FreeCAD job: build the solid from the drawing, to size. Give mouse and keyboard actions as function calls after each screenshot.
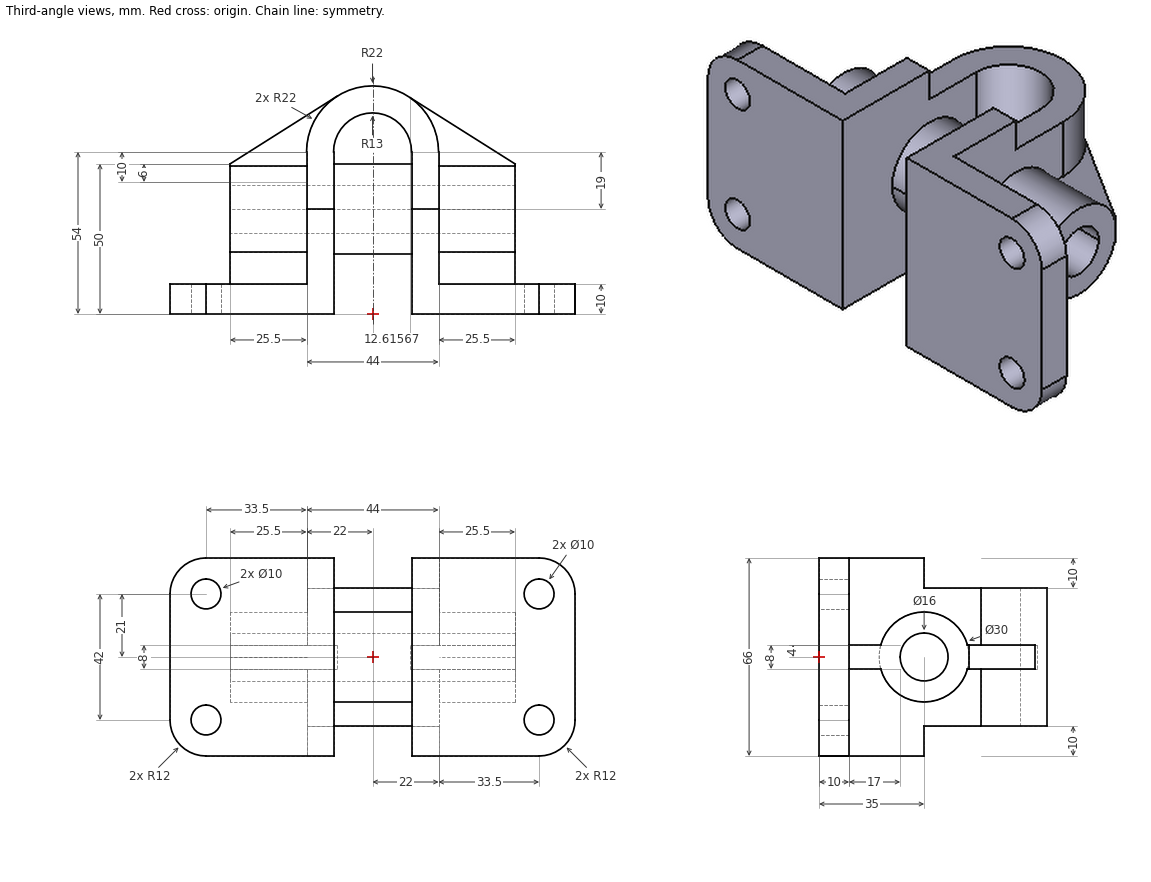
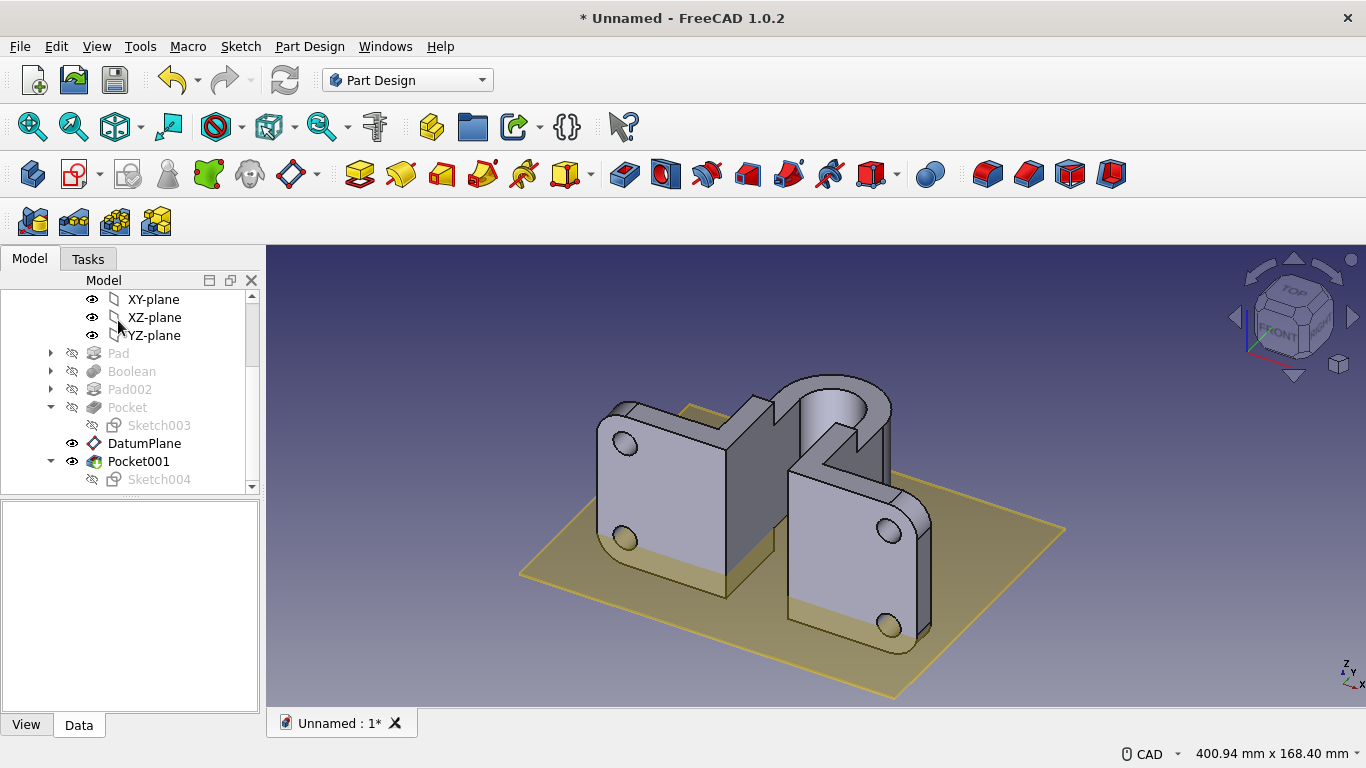
click(117, 443)
key(space)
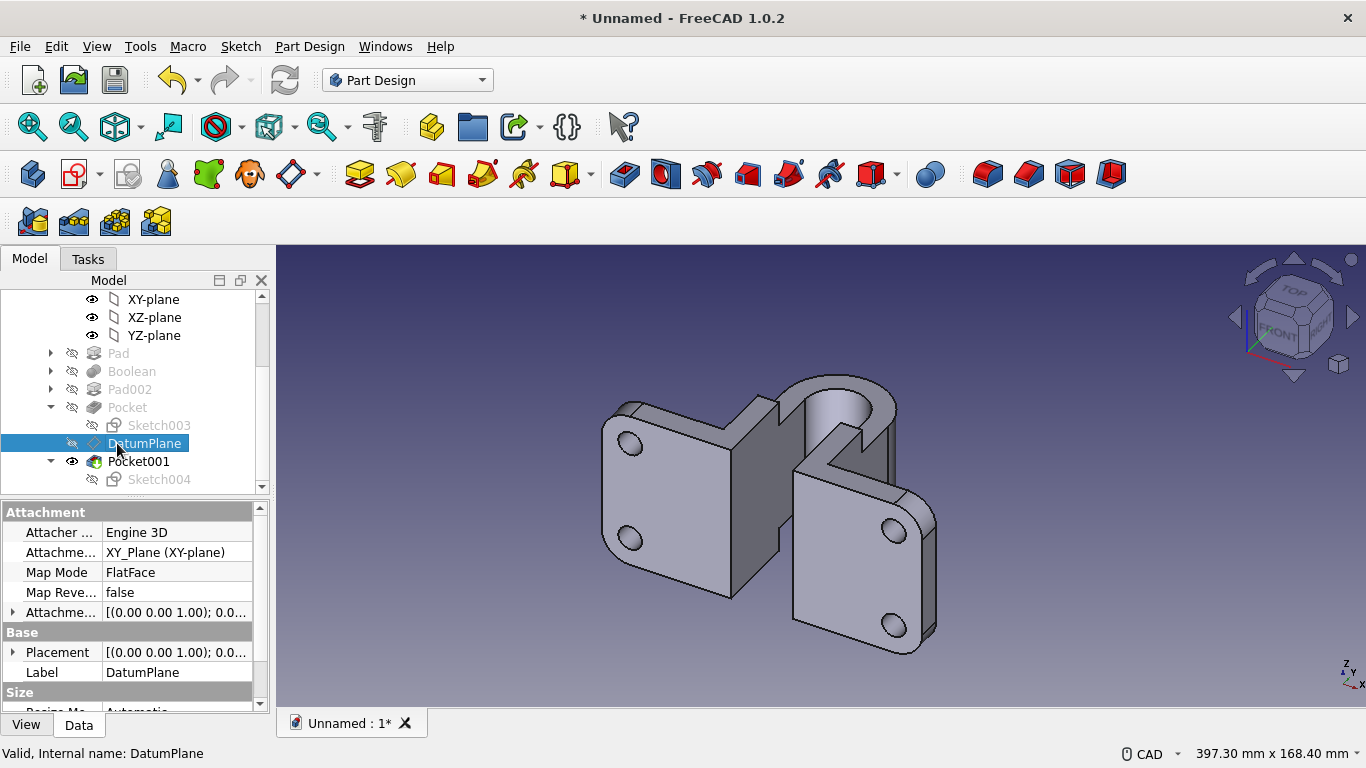
key(6)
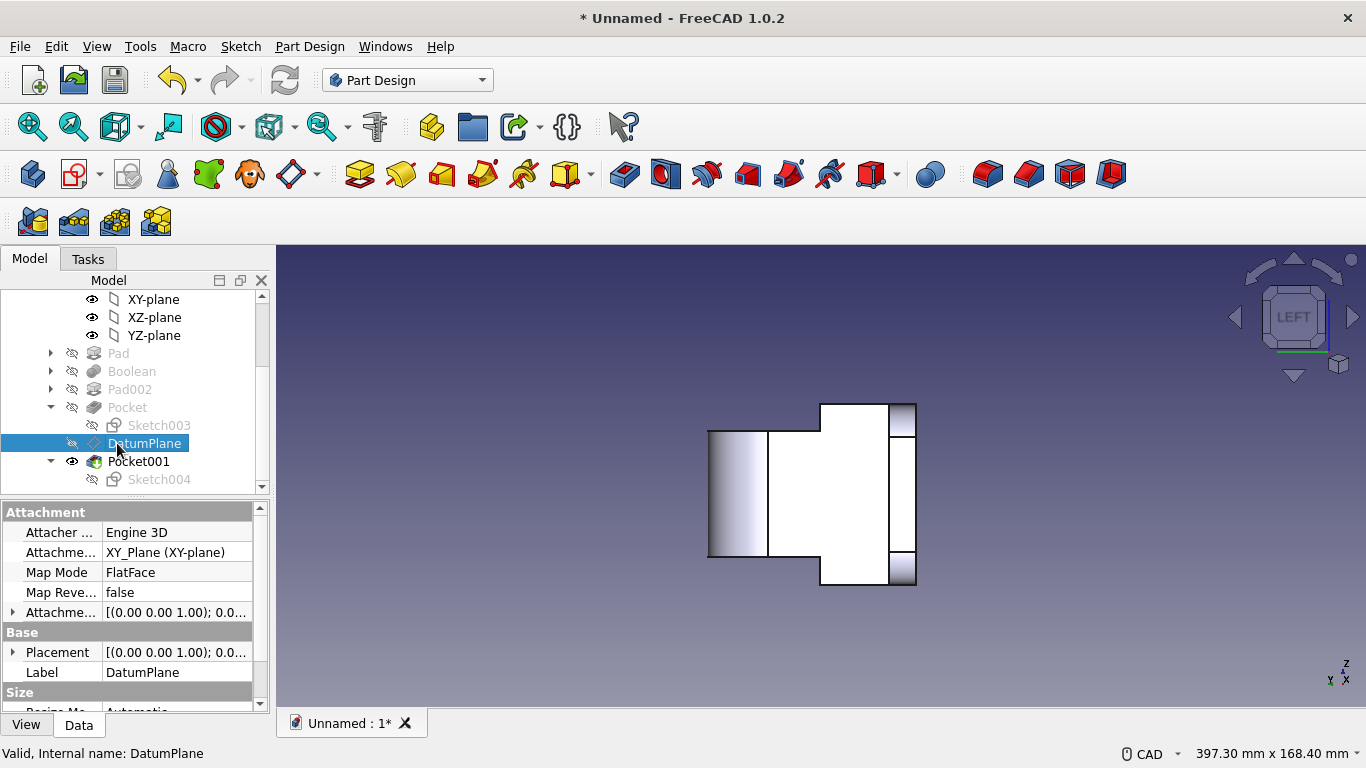
click(33, 128)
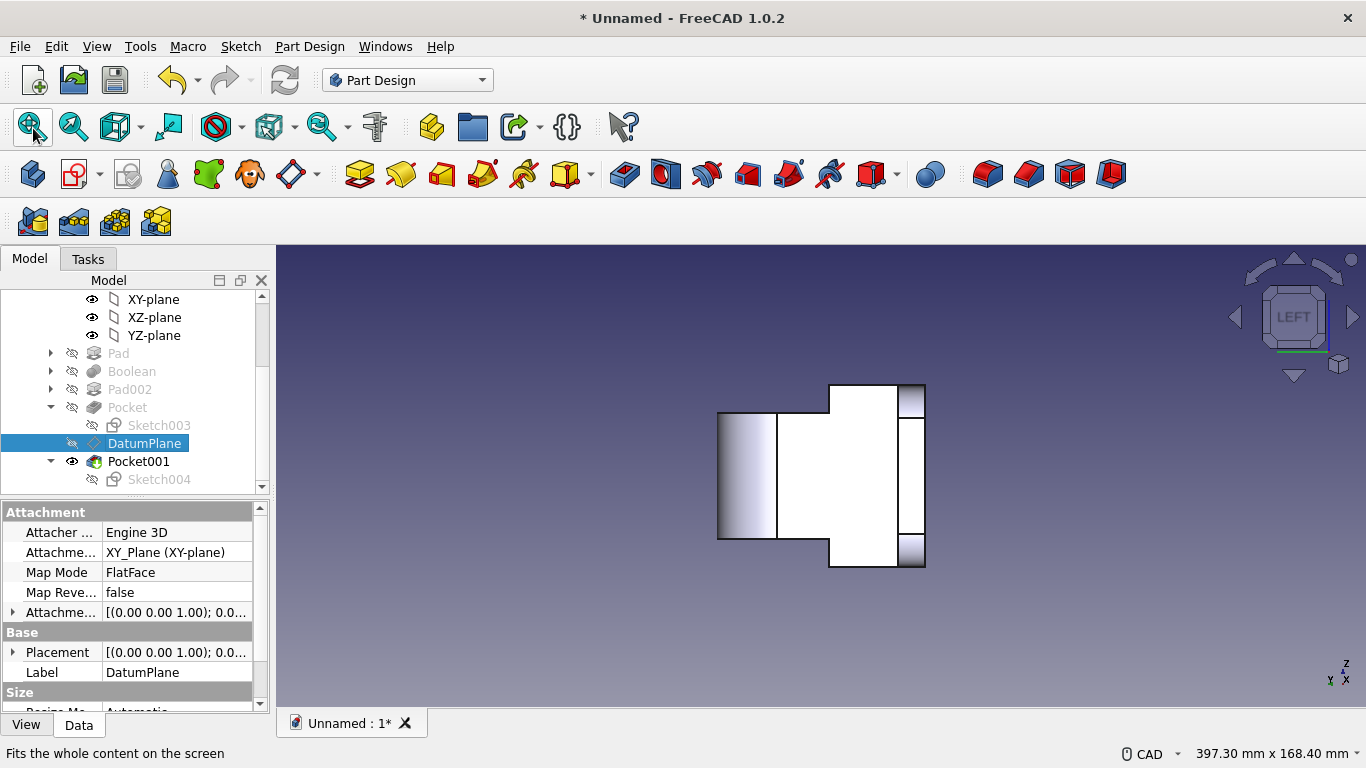
click(837, 475)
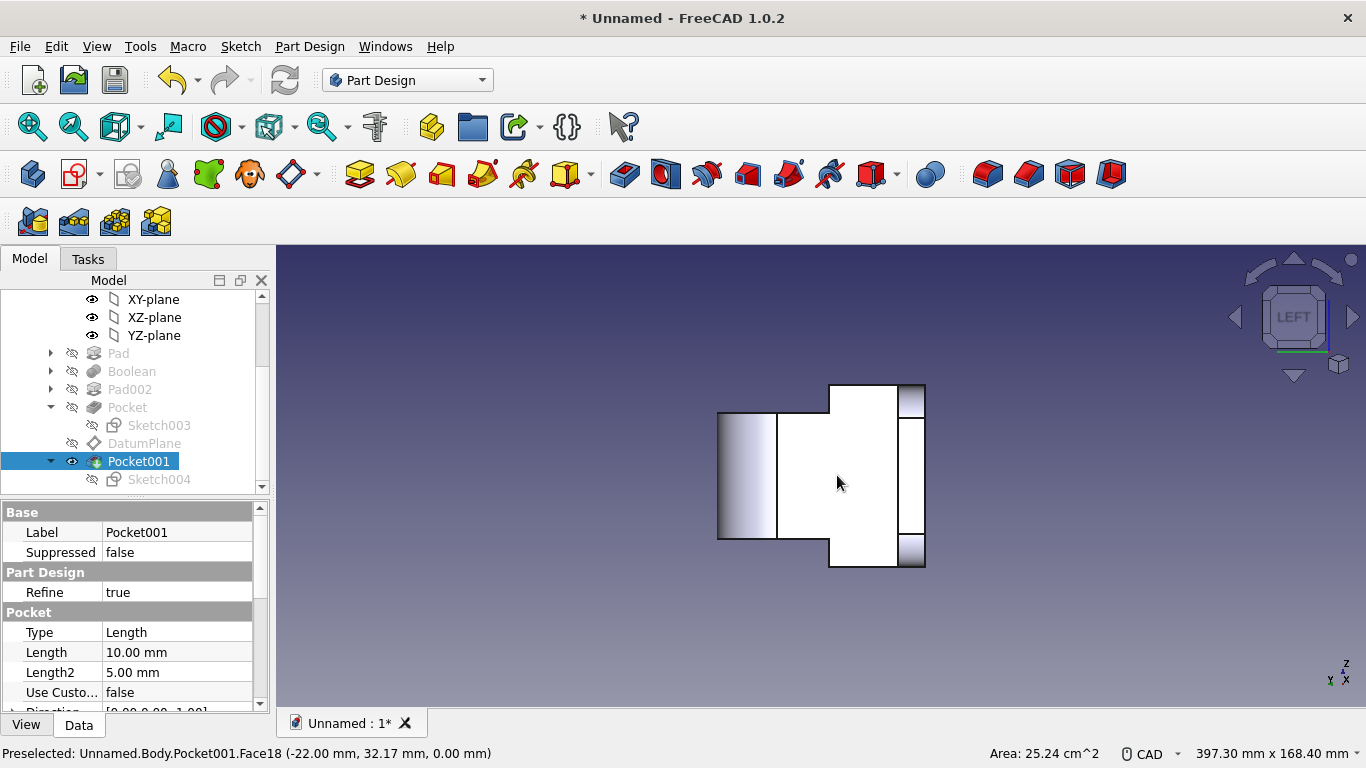
click(74, 174)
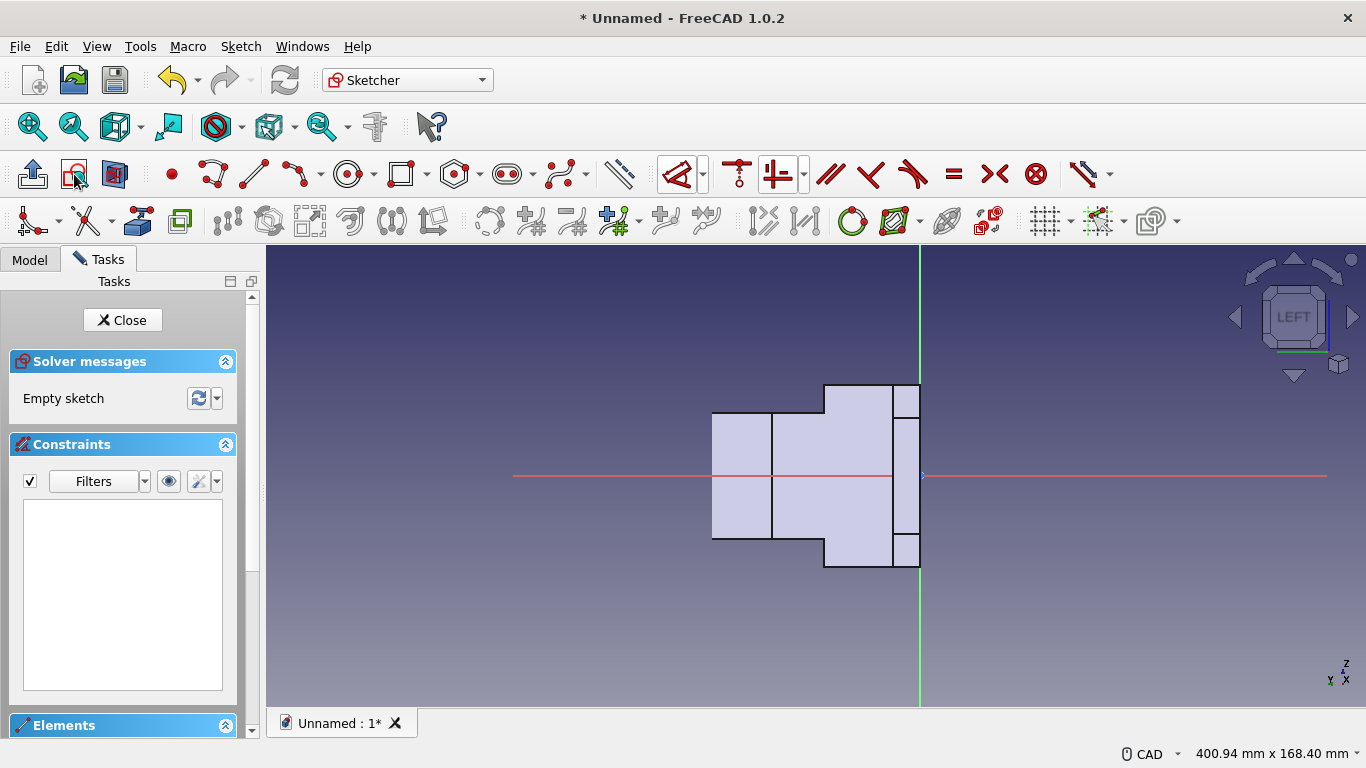
scroll(897, 476, up, 6)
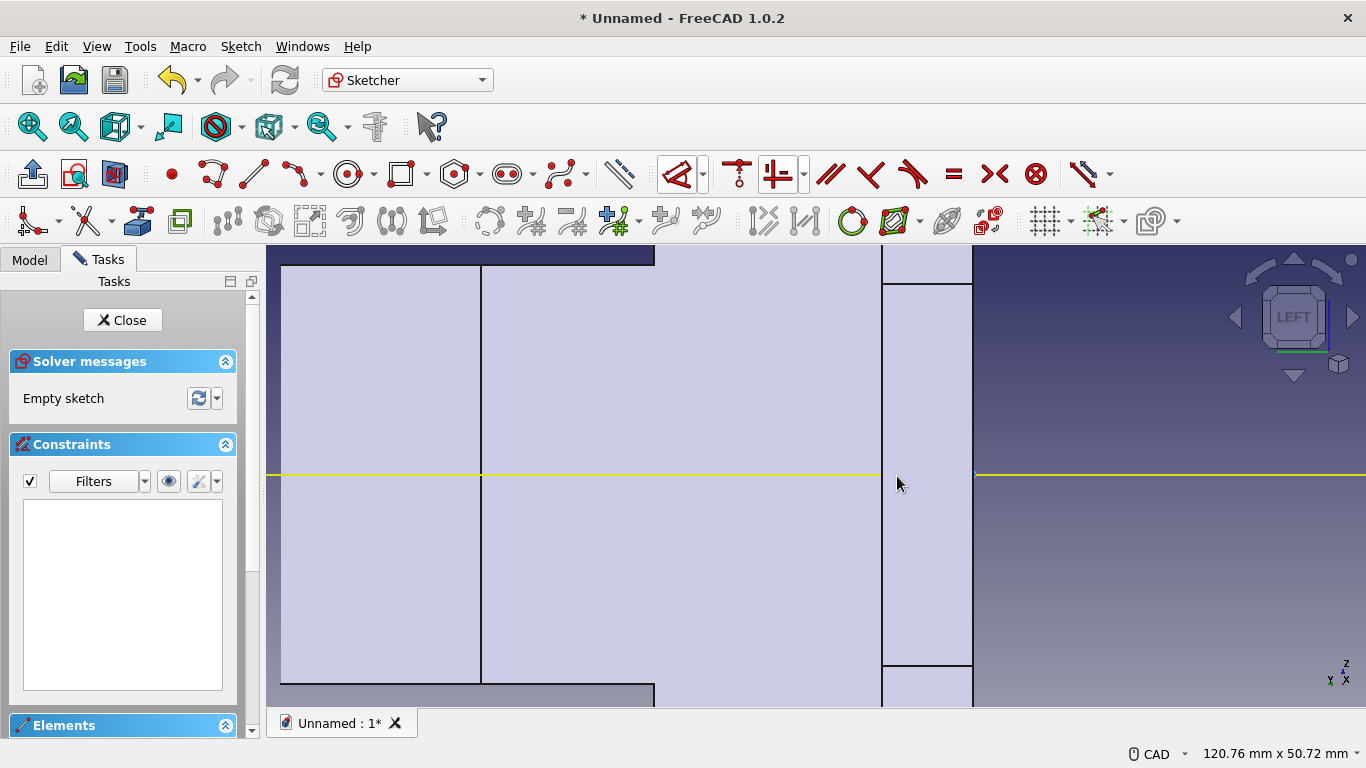
click(348, 174)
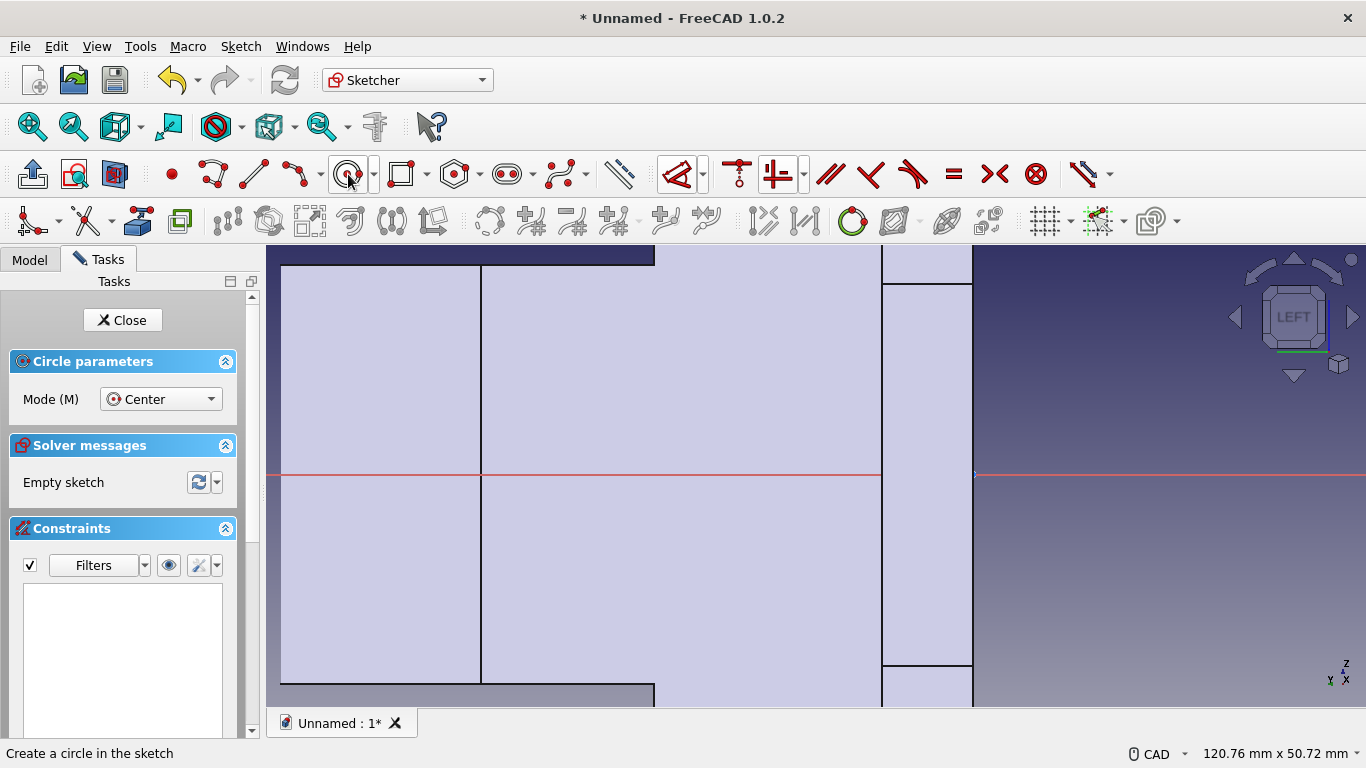
click(654, 475)
move(751, 378)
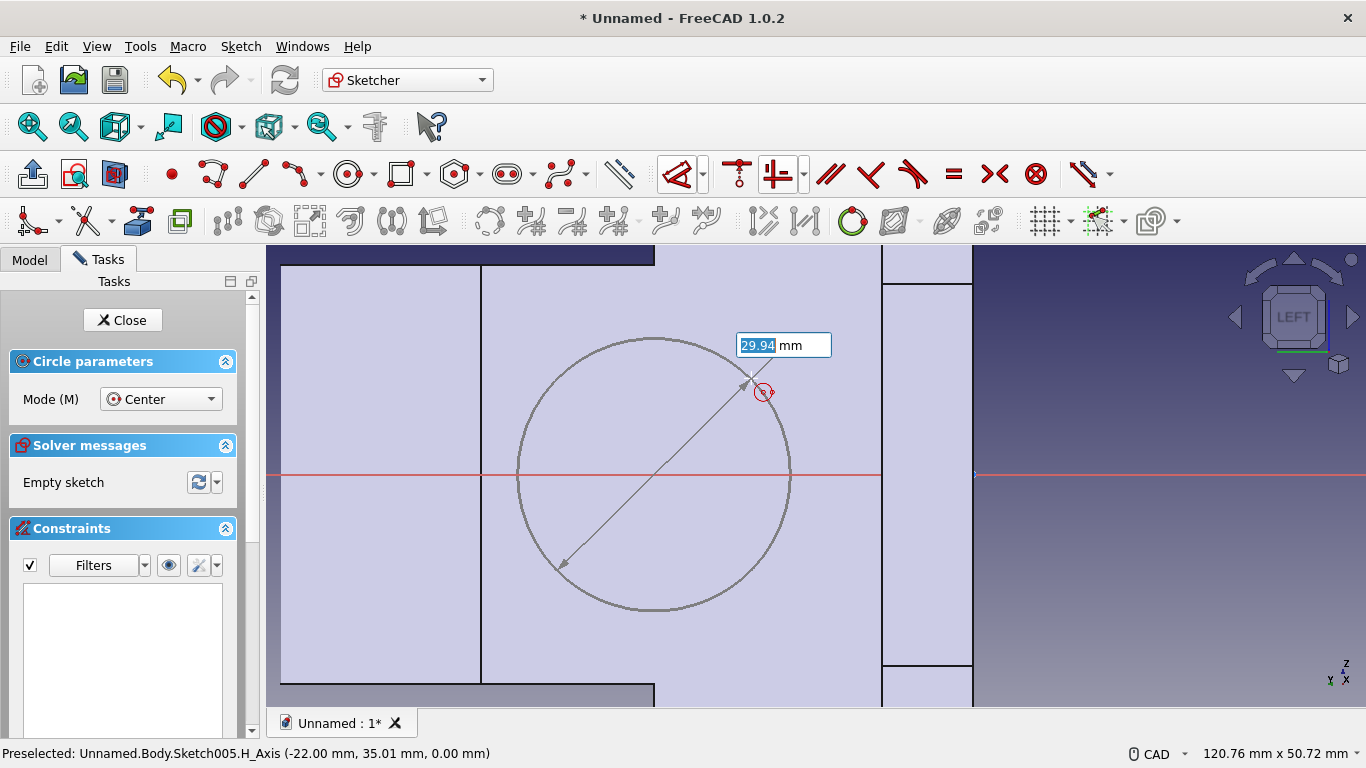
text(30)
key(Return)